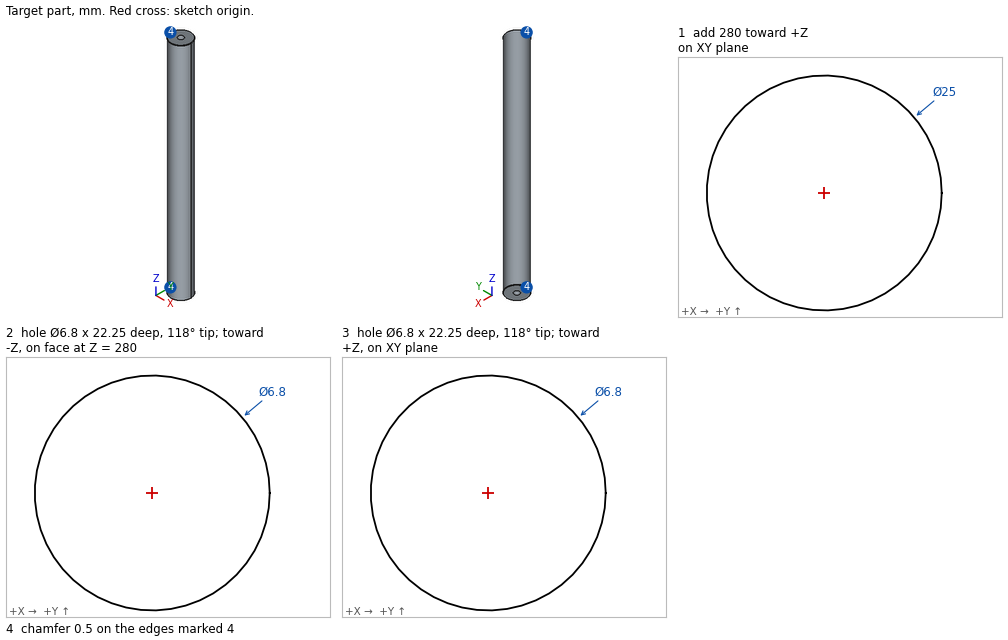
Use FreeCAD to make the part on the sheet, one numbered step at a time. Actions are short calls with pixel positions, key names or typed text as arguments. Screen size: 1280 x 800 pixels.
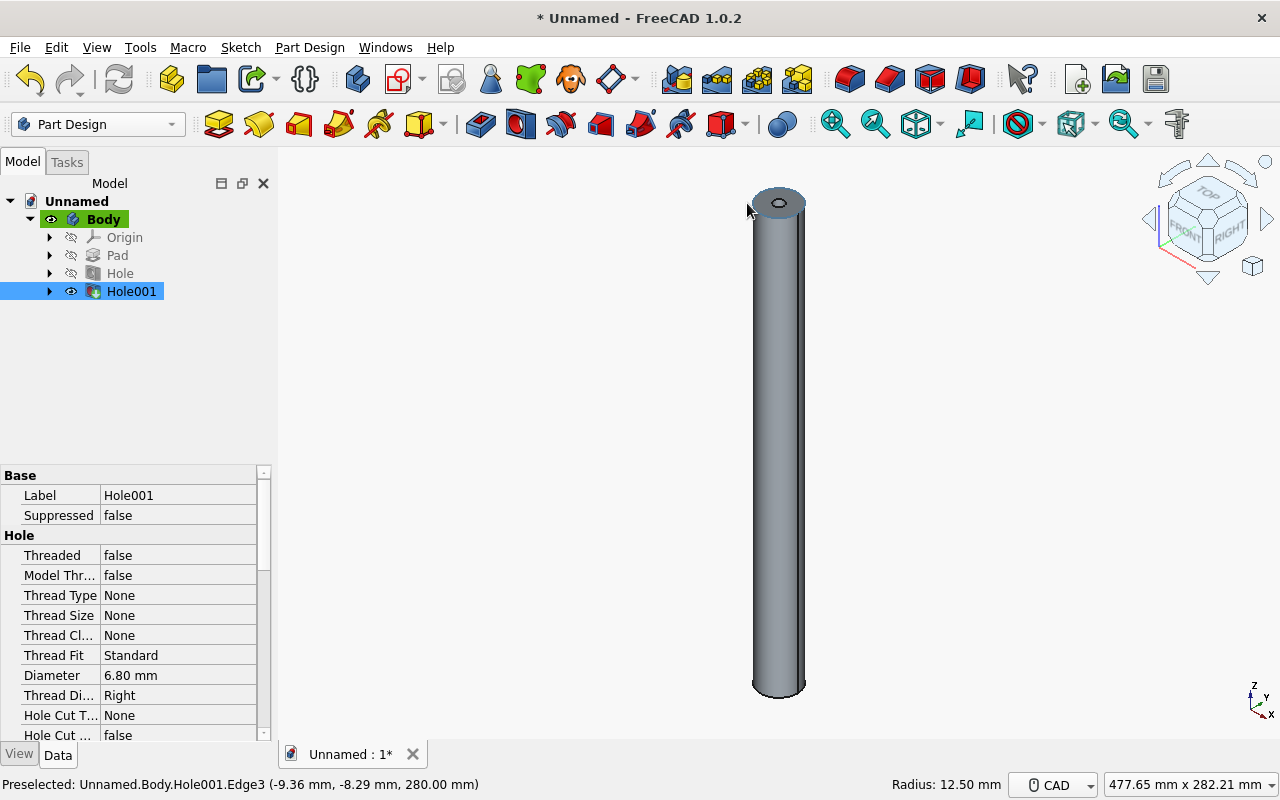
click(756, 689, ctrl)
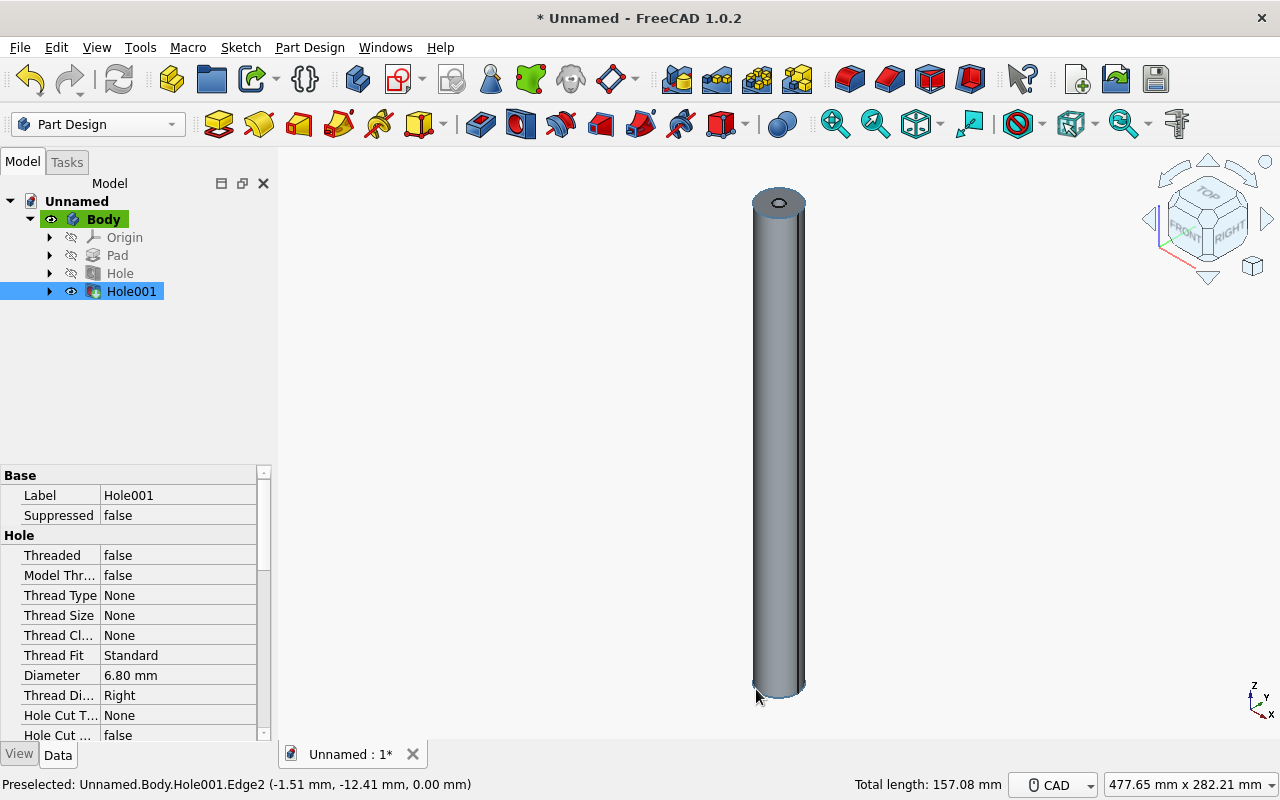
click(890, 80)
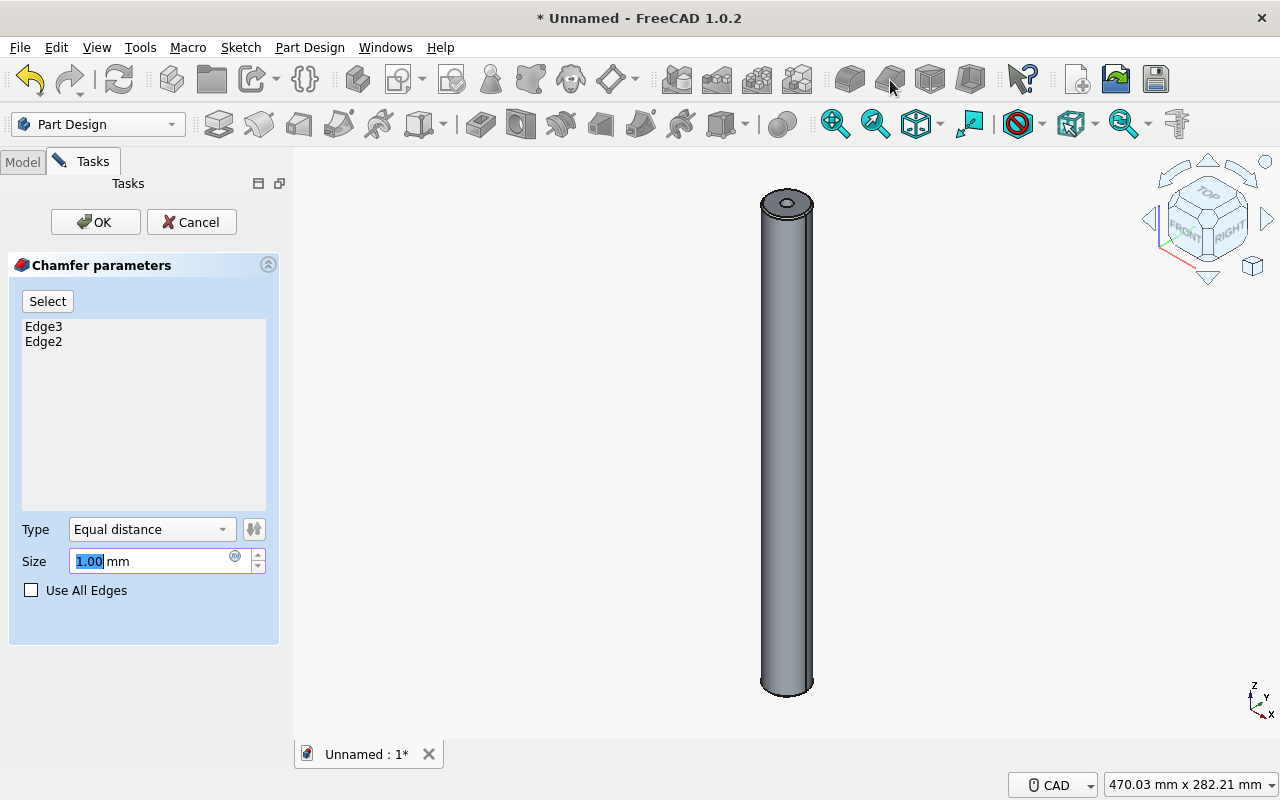
text(0.5)
key(Tab)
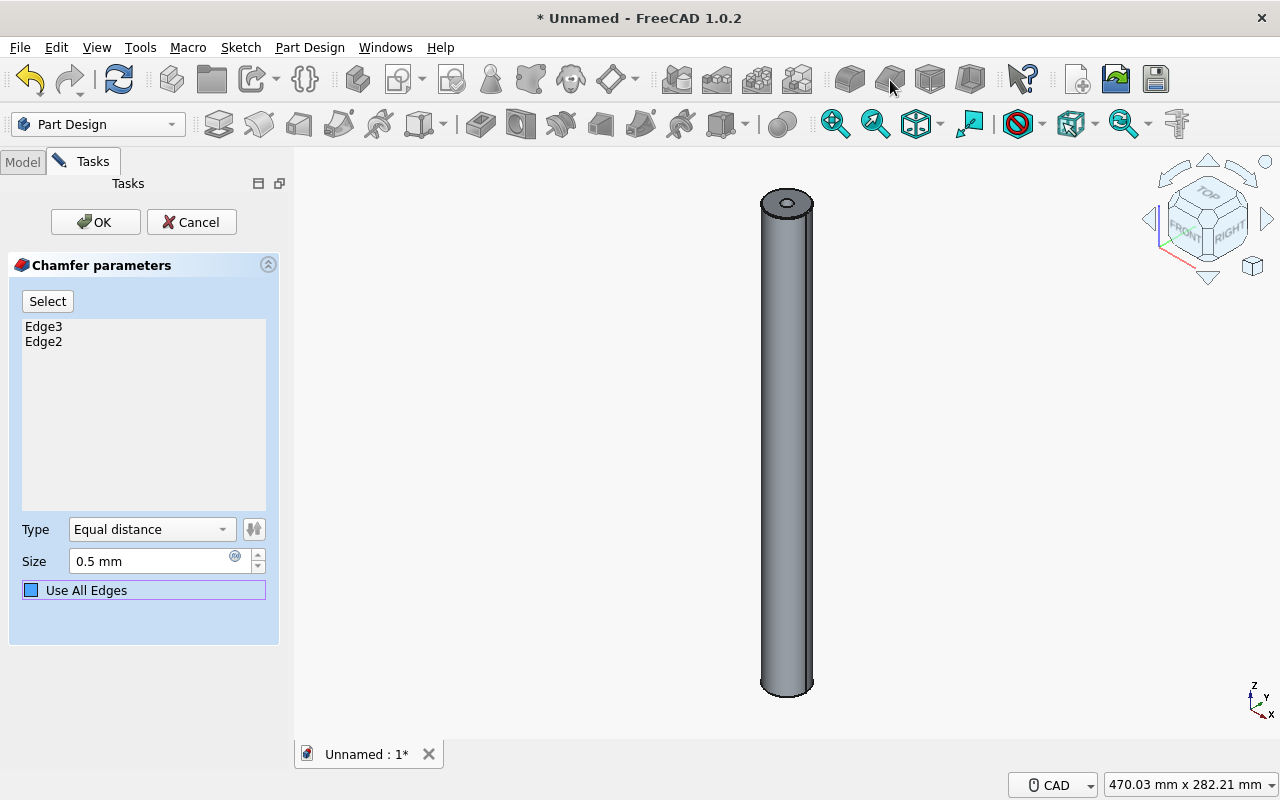
click(96, 222)